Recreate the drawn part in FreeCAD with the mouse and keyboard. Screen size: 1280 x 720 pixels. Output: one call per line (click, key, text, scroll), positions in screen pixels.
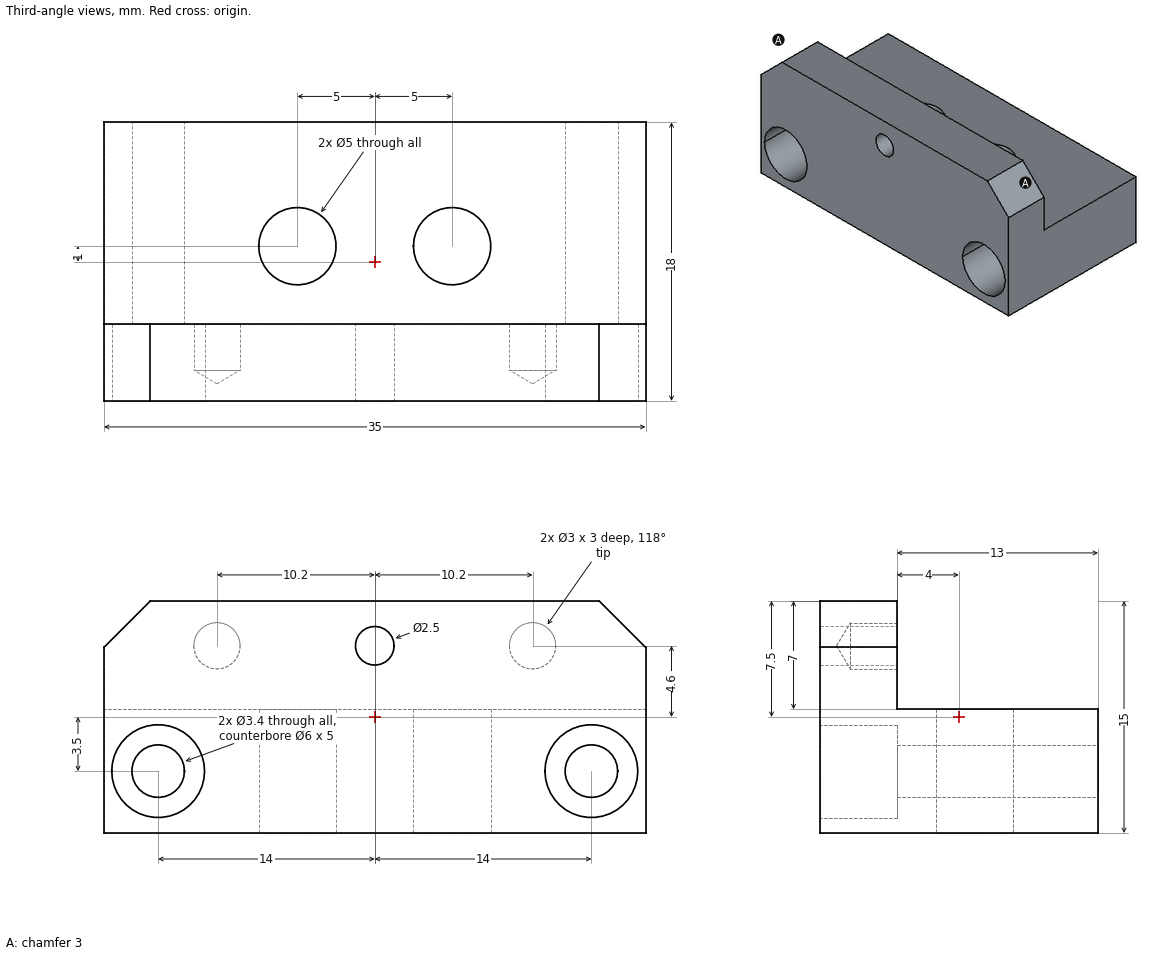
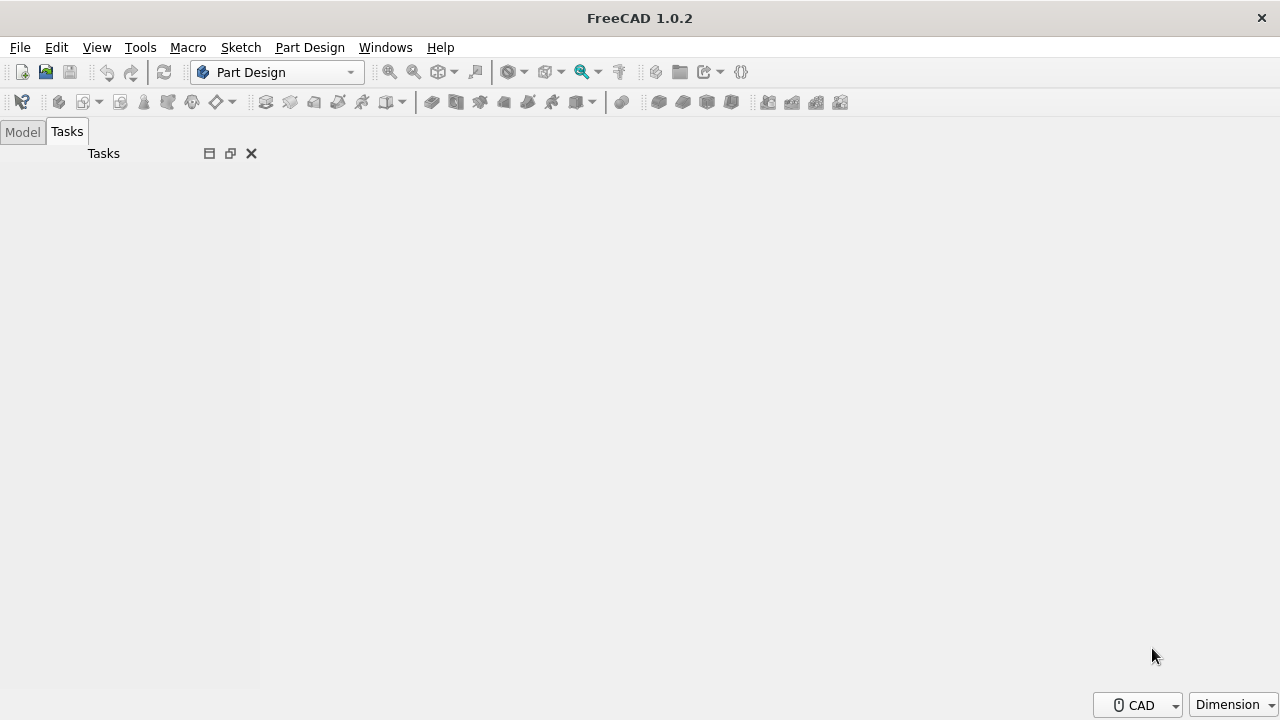
key(ctrl+n)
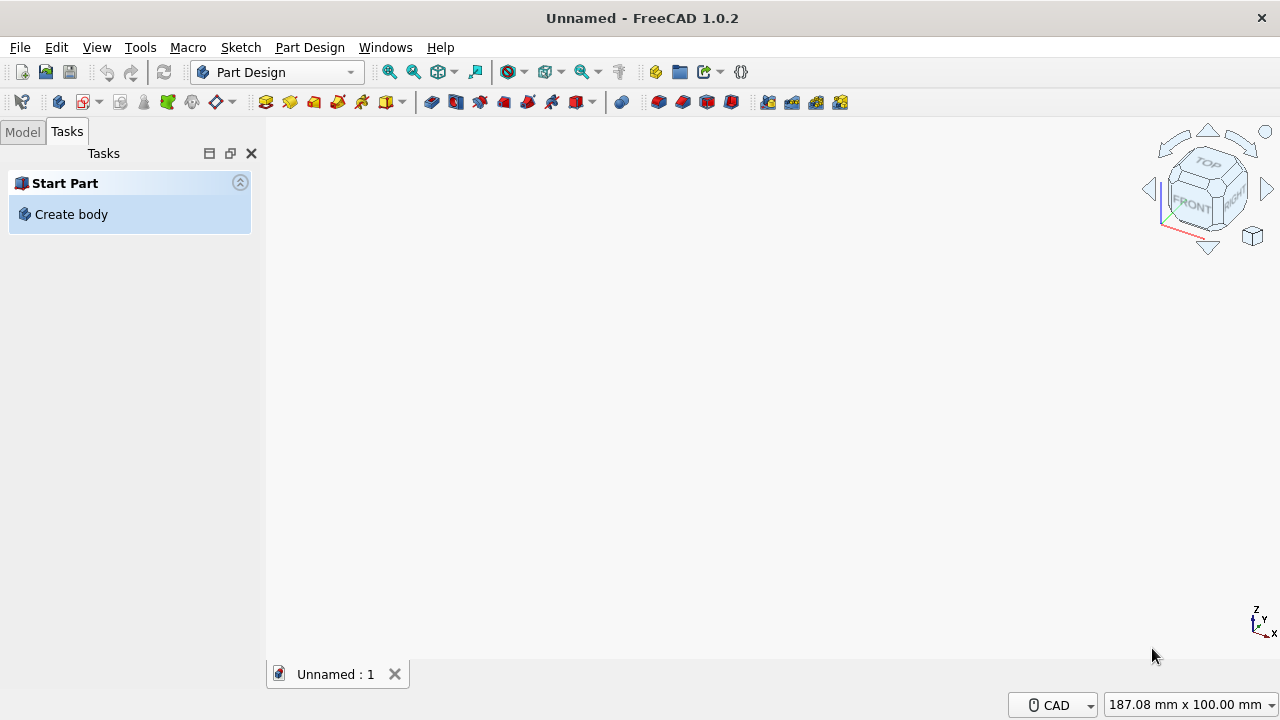
click(84, 102)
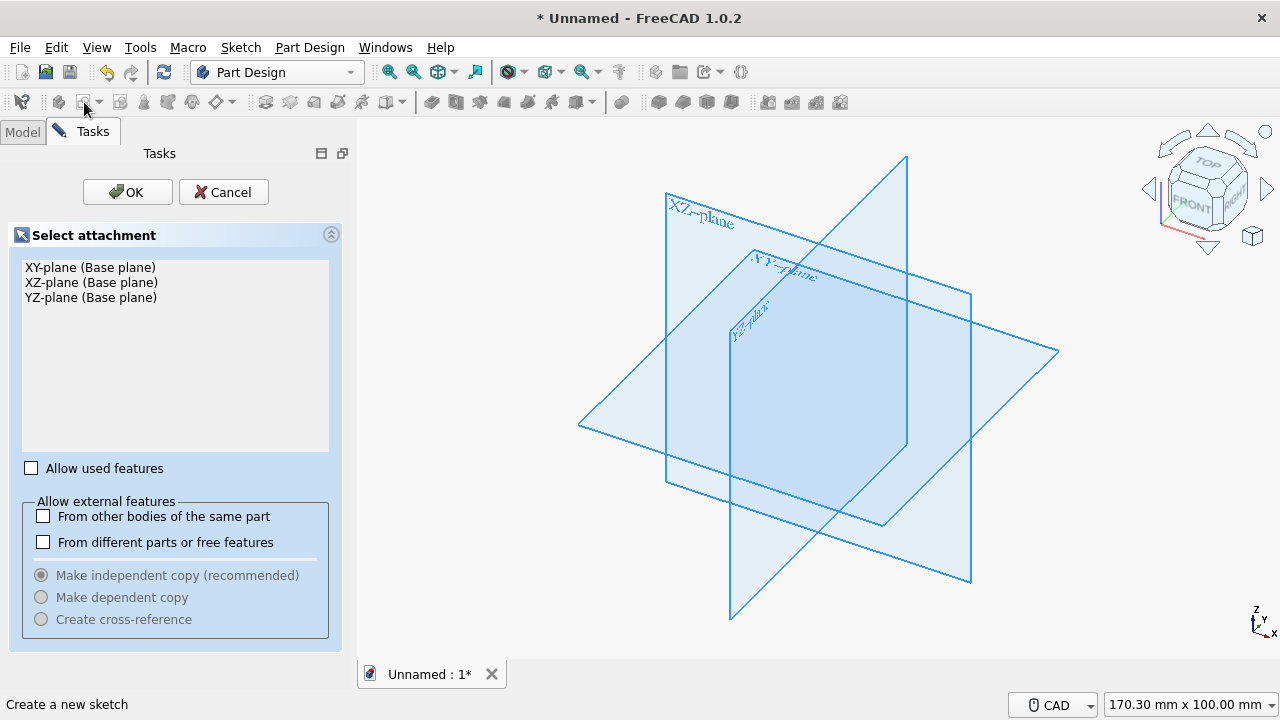
click(82, 268)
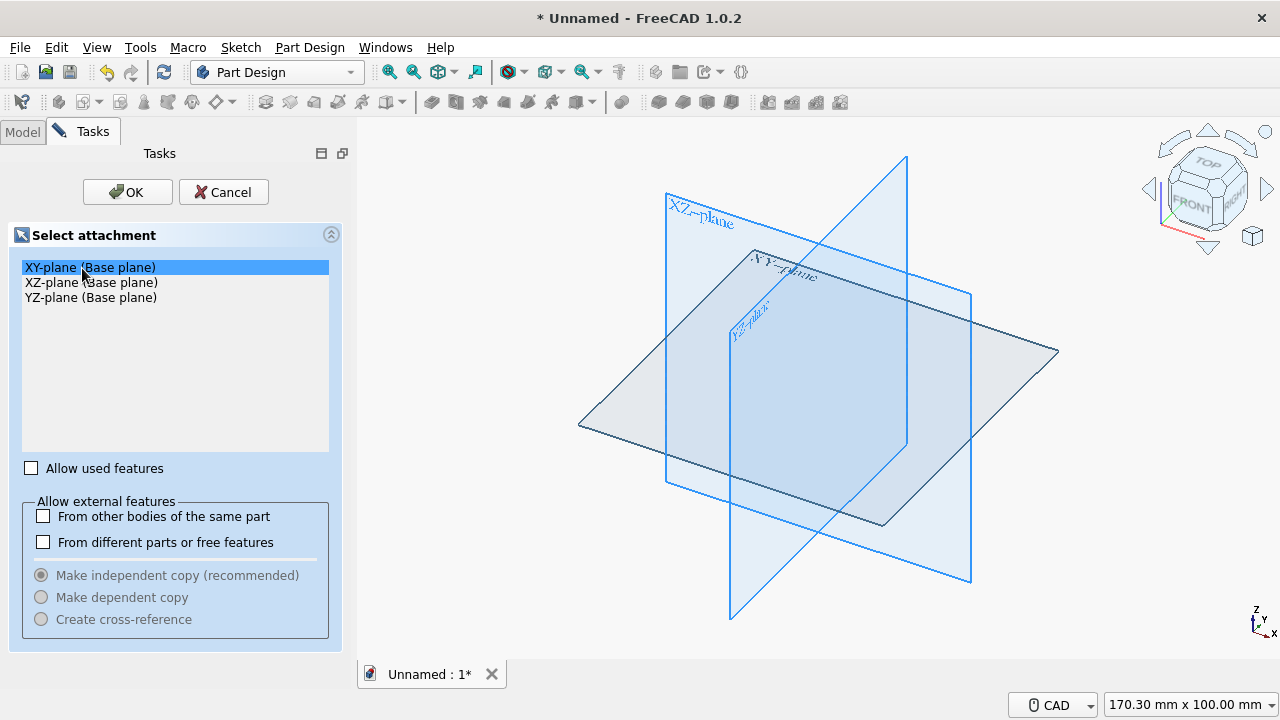
click(128, 192)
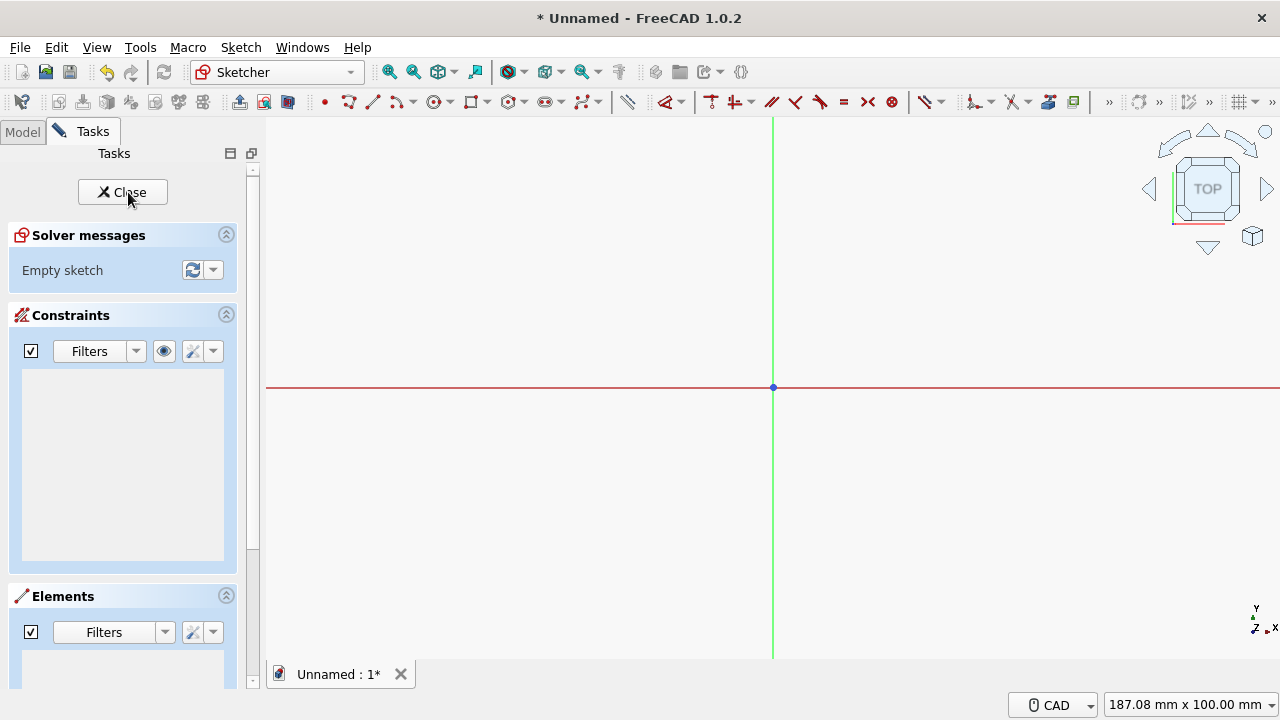
scroll(803, 388, up, 6)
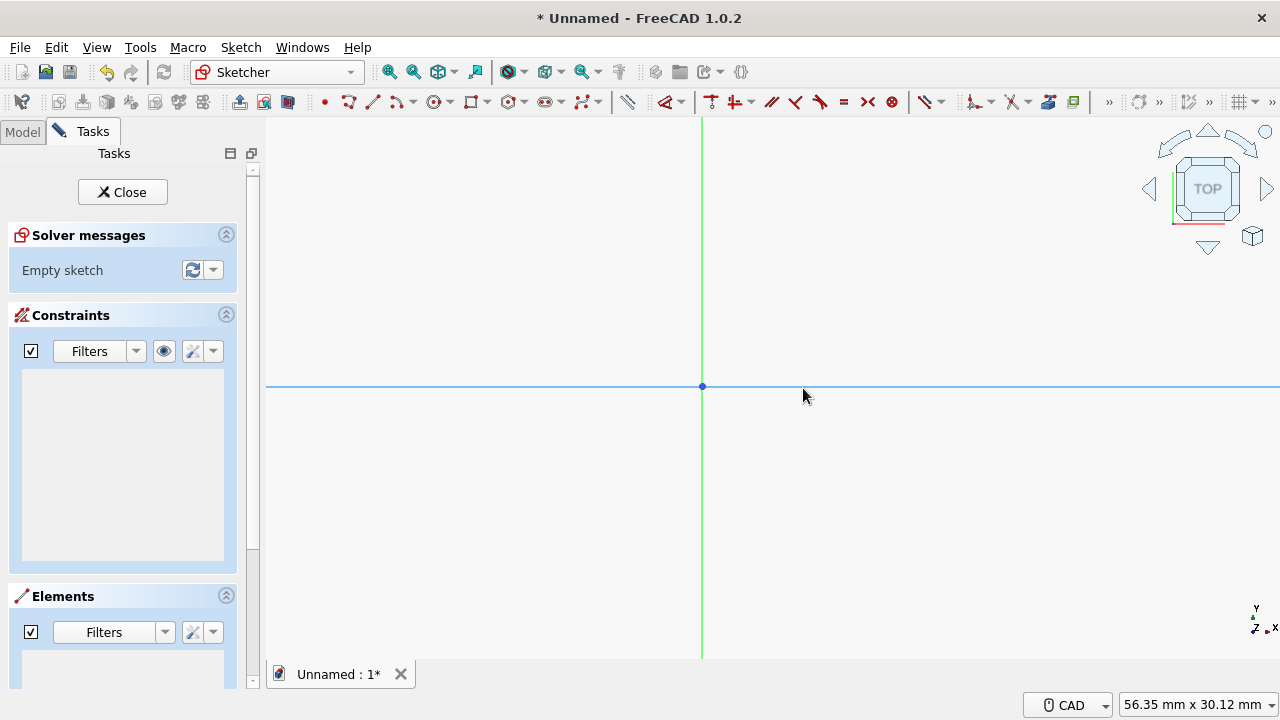
key(g)
key(v)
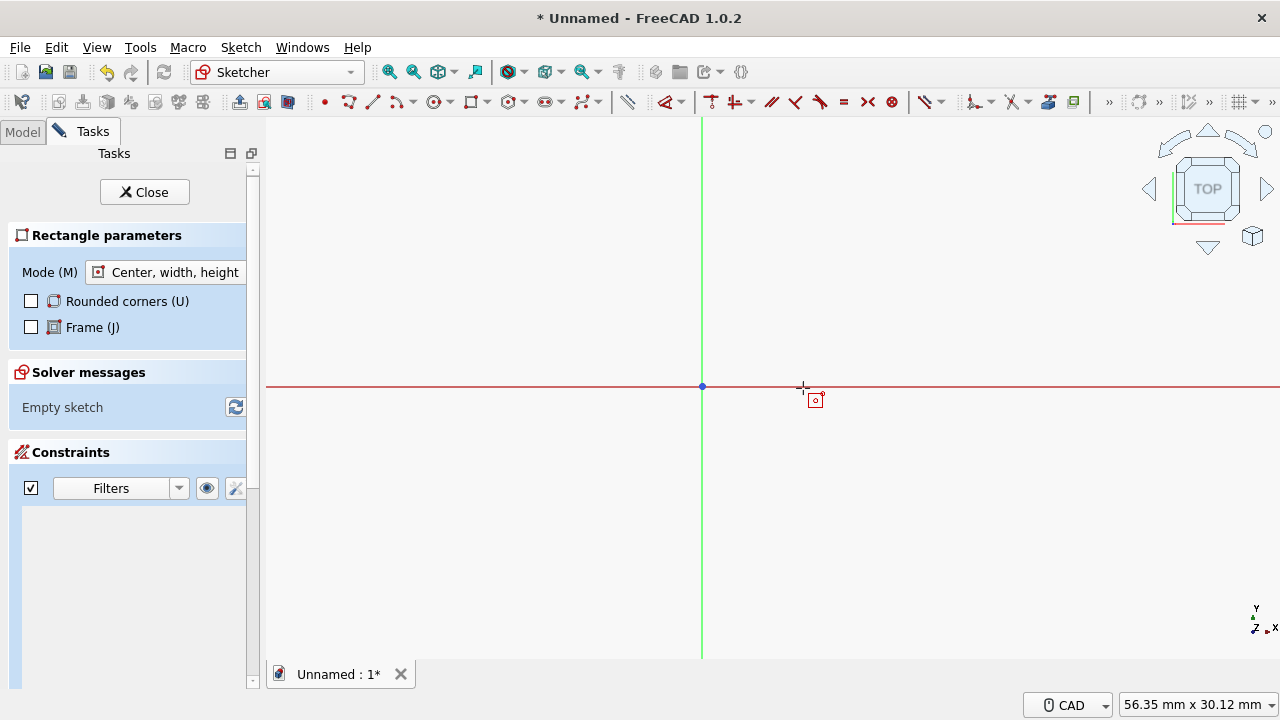
click(702, 387)
click(1017, 225)
key(Escape)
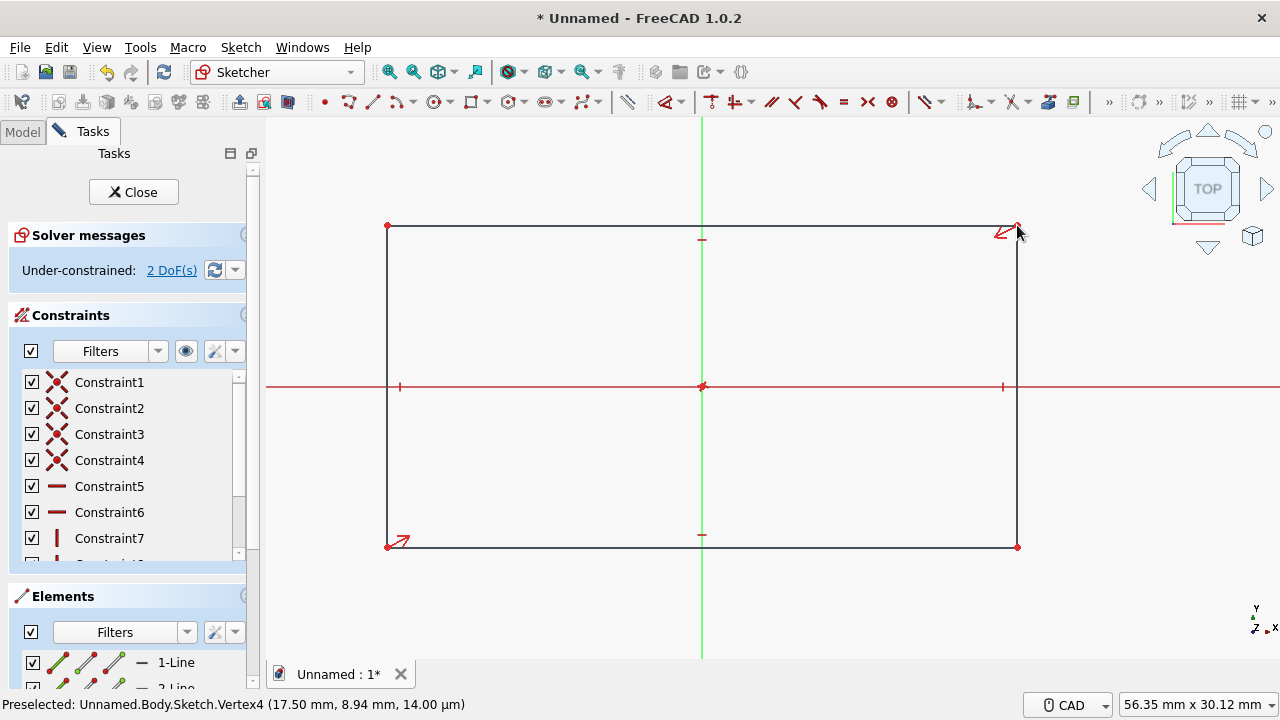
key(d)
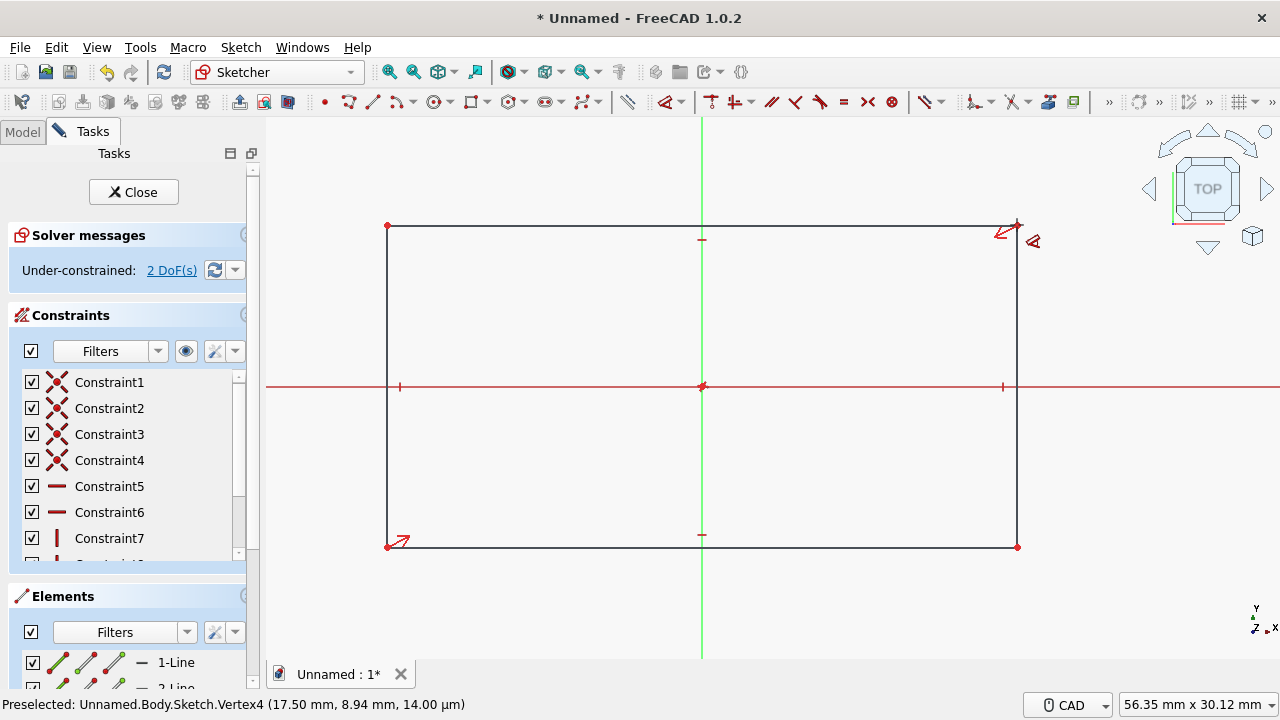
click(576, 548)
click(557, 582)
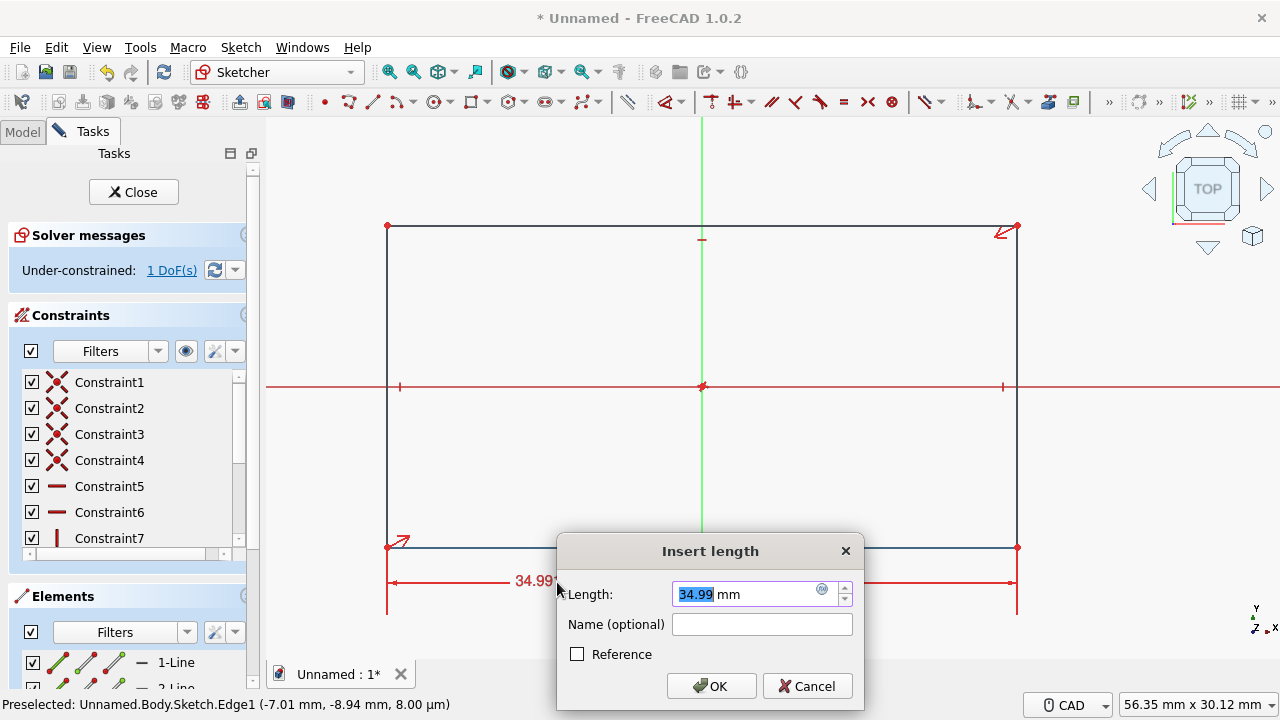
text(35)
key(Return)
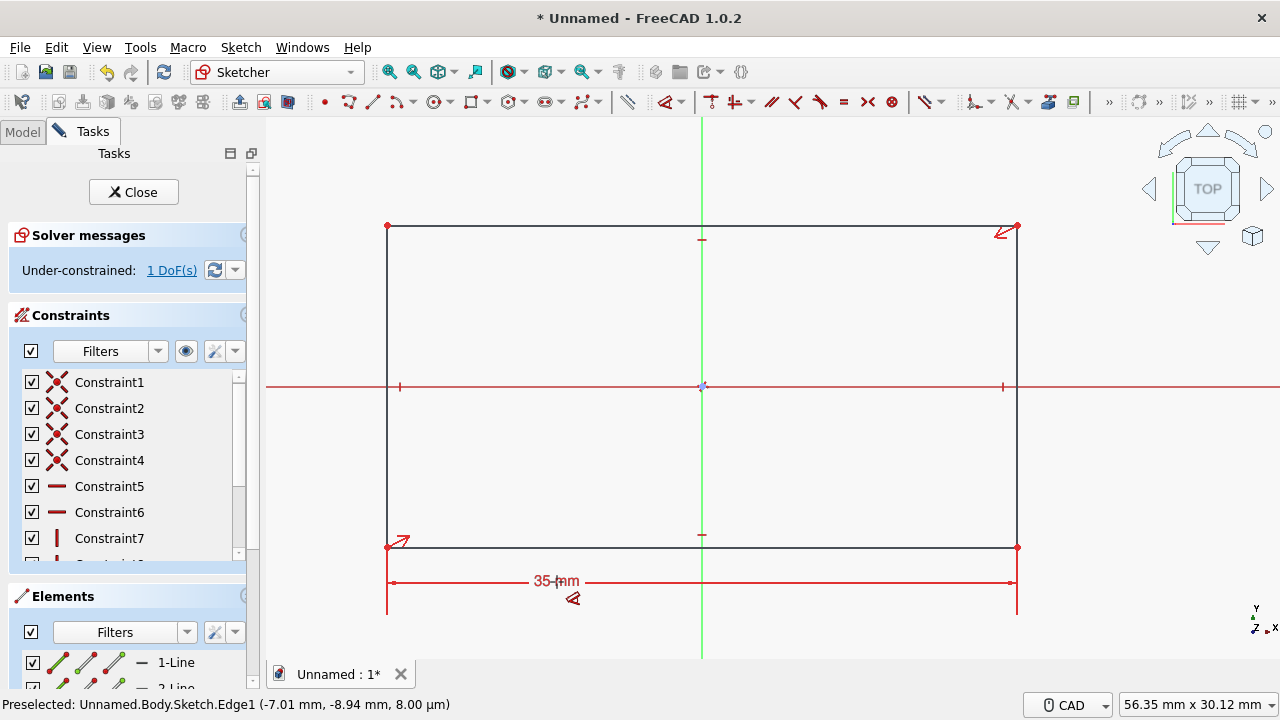
click(1017, 451)
click(1051, 313)